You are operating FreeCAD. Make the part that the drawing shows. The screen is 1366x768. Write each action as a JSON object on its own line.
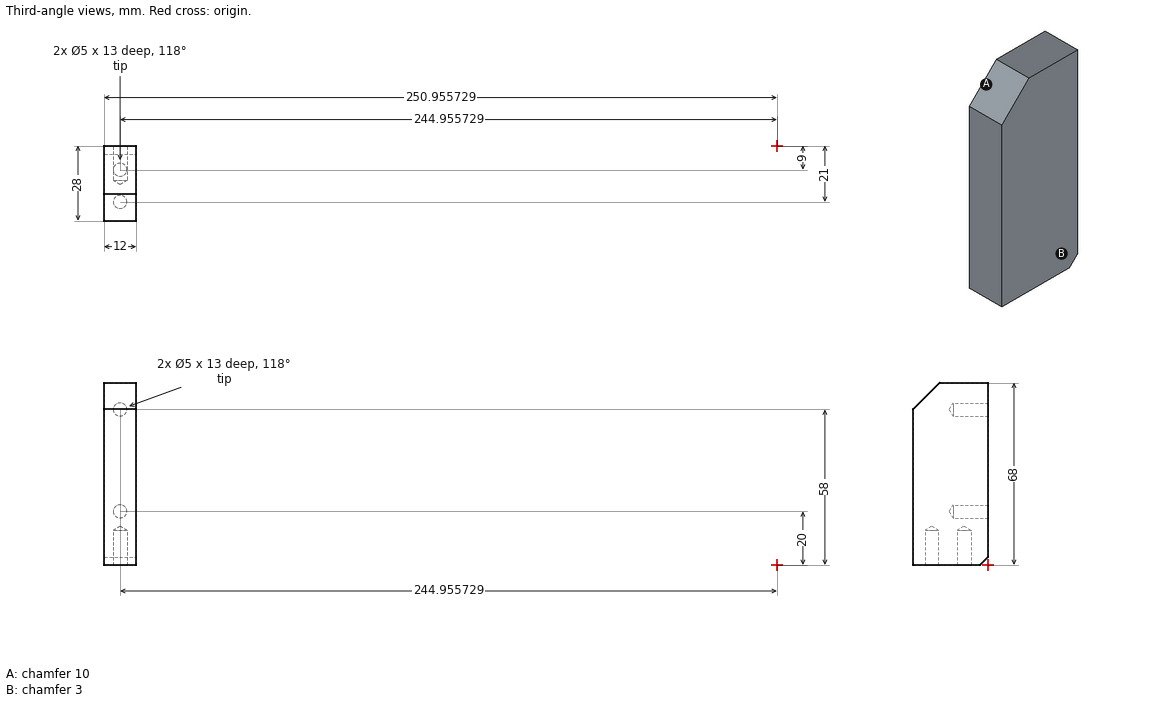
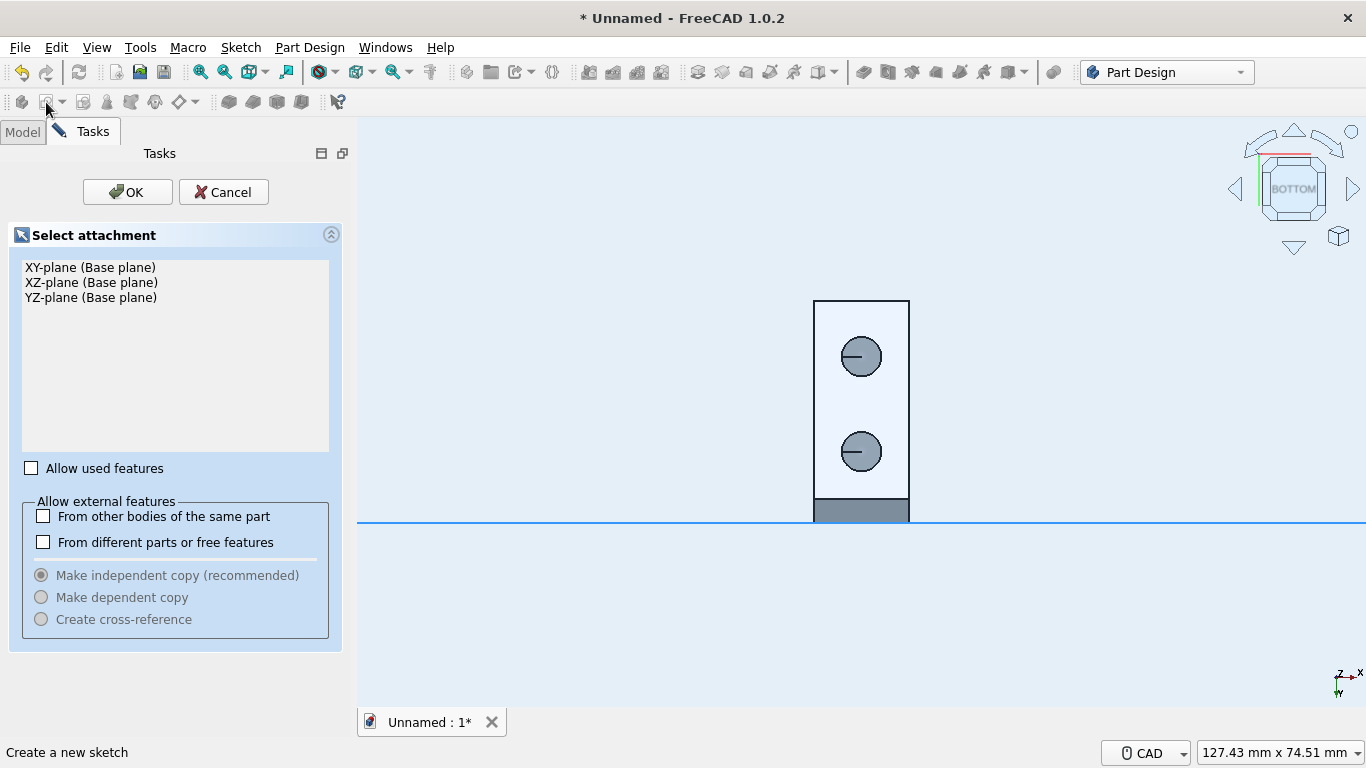
{"action": "left_click", "coordinate": [82, 282]}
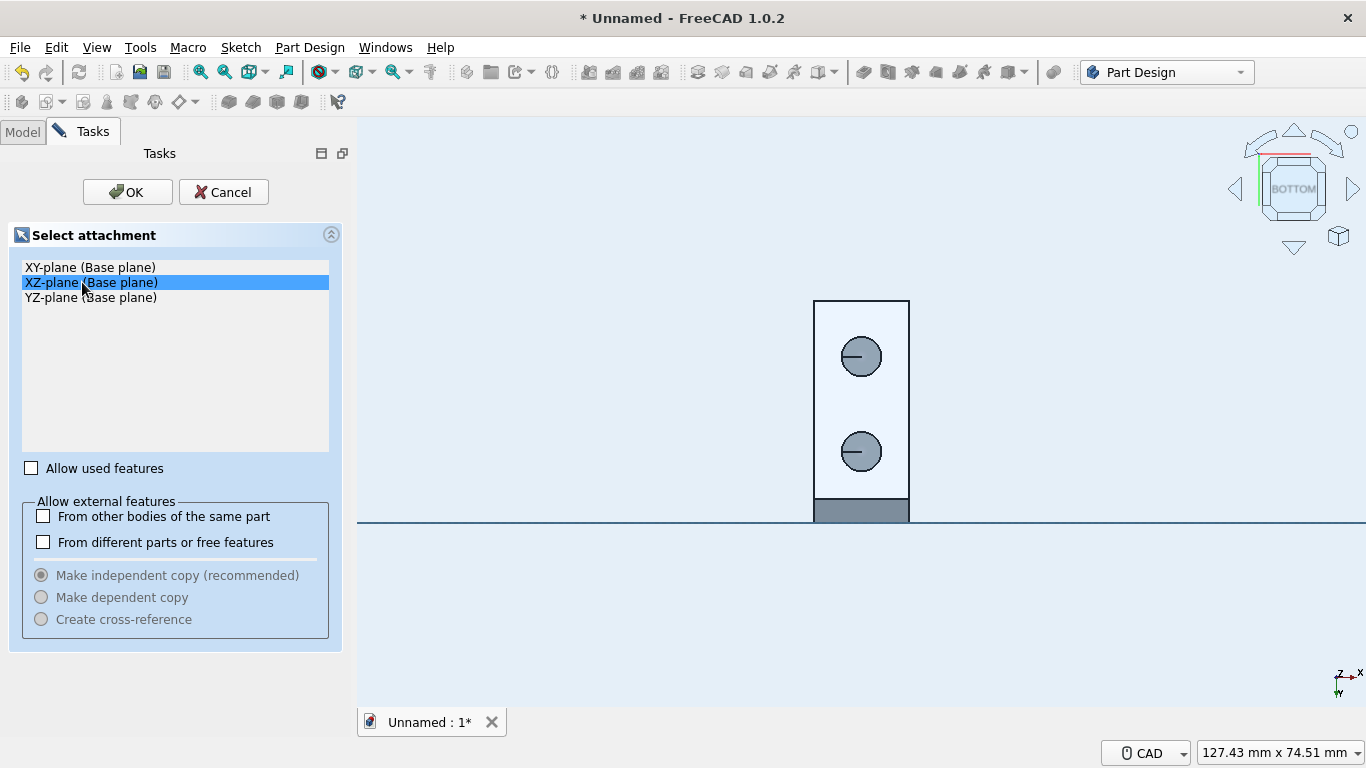
{"action": "left_click", "coordinate": [128, 192]}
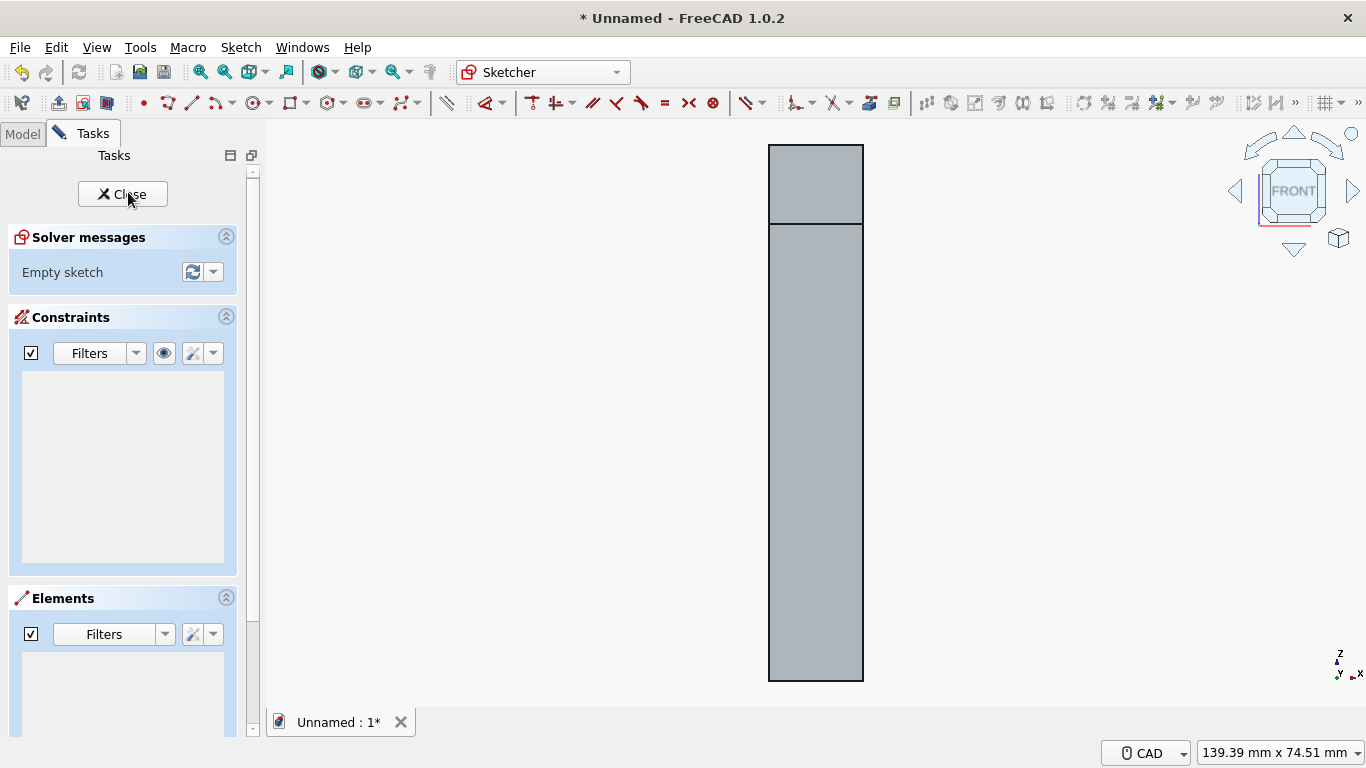
{"action": "left_click", "coordinate": [108, 104]}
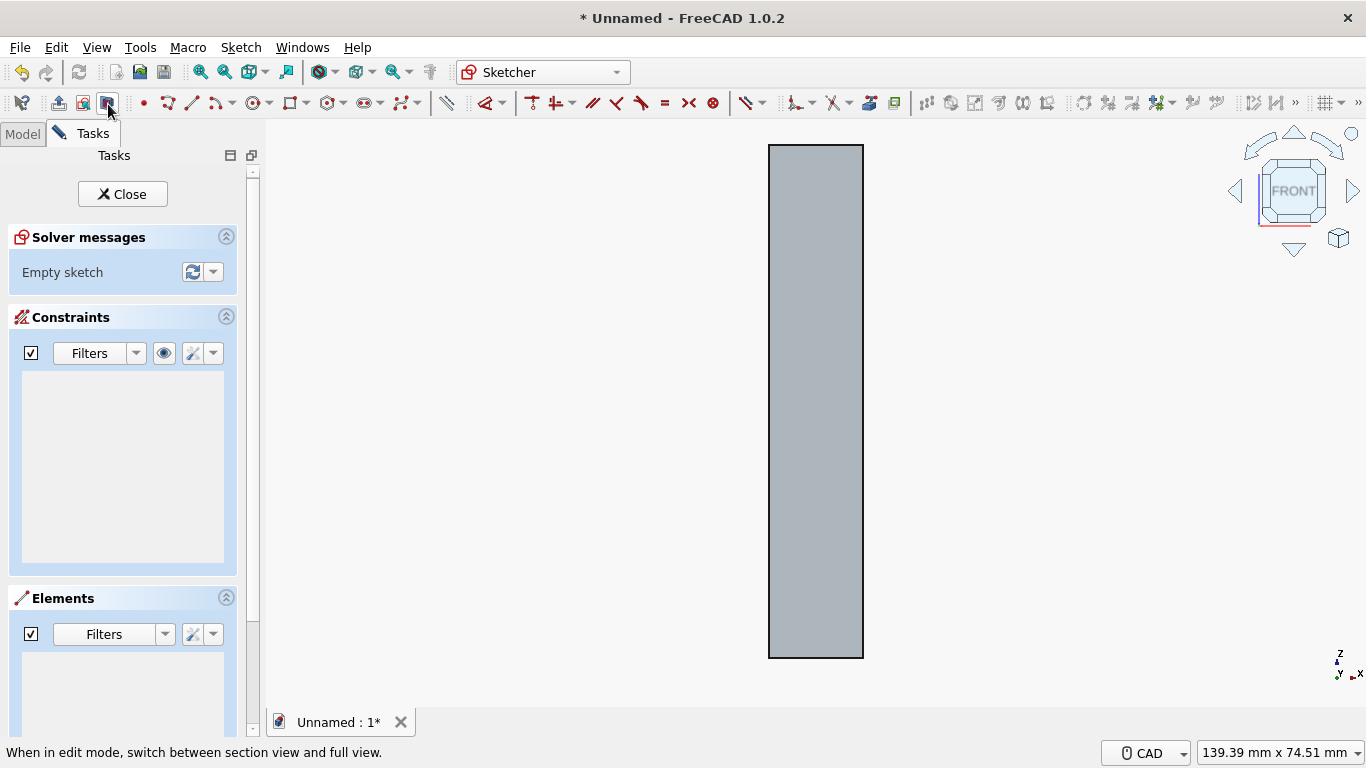
{"action": "left_click", "coordinate": [254, 104]}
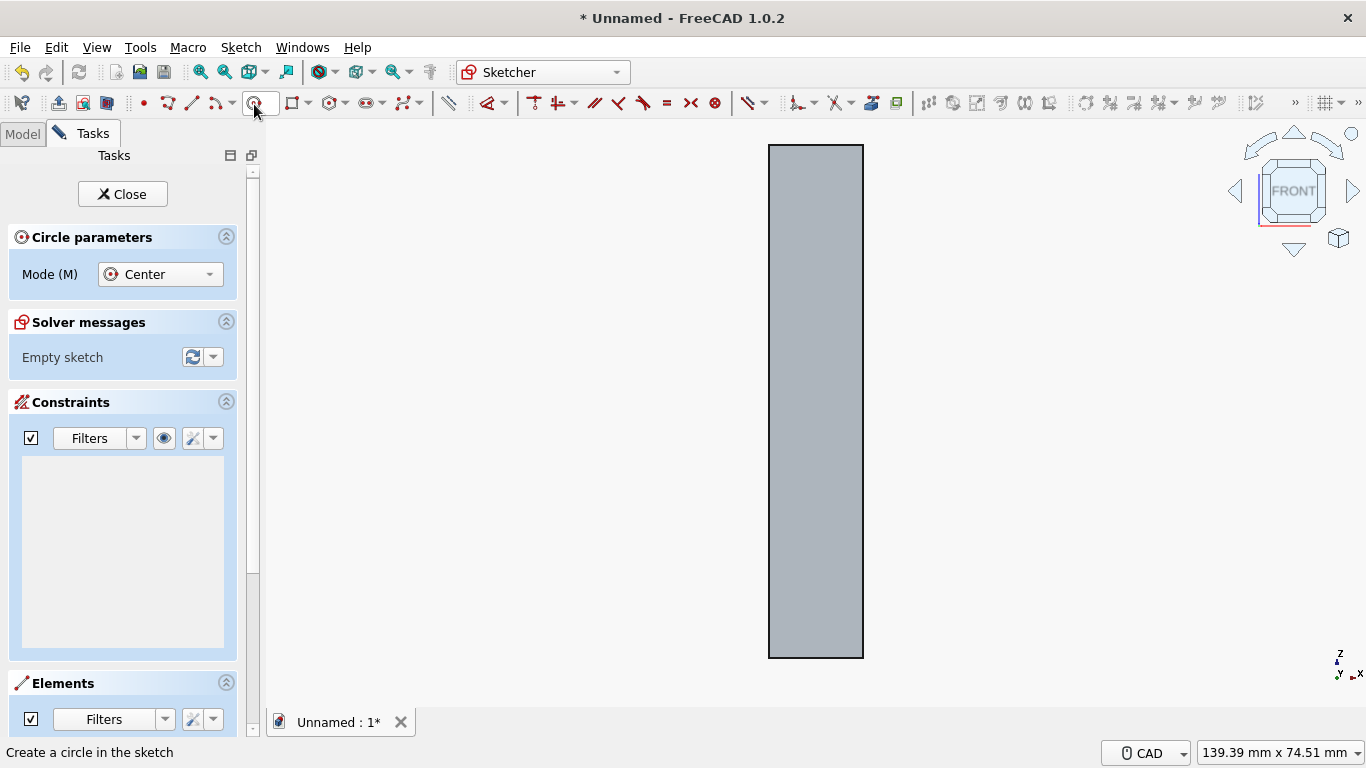
{"action": "left_click", "coordinate": [816, 224]}
{"action": "mouse_move", "coordinate": [830, 210]}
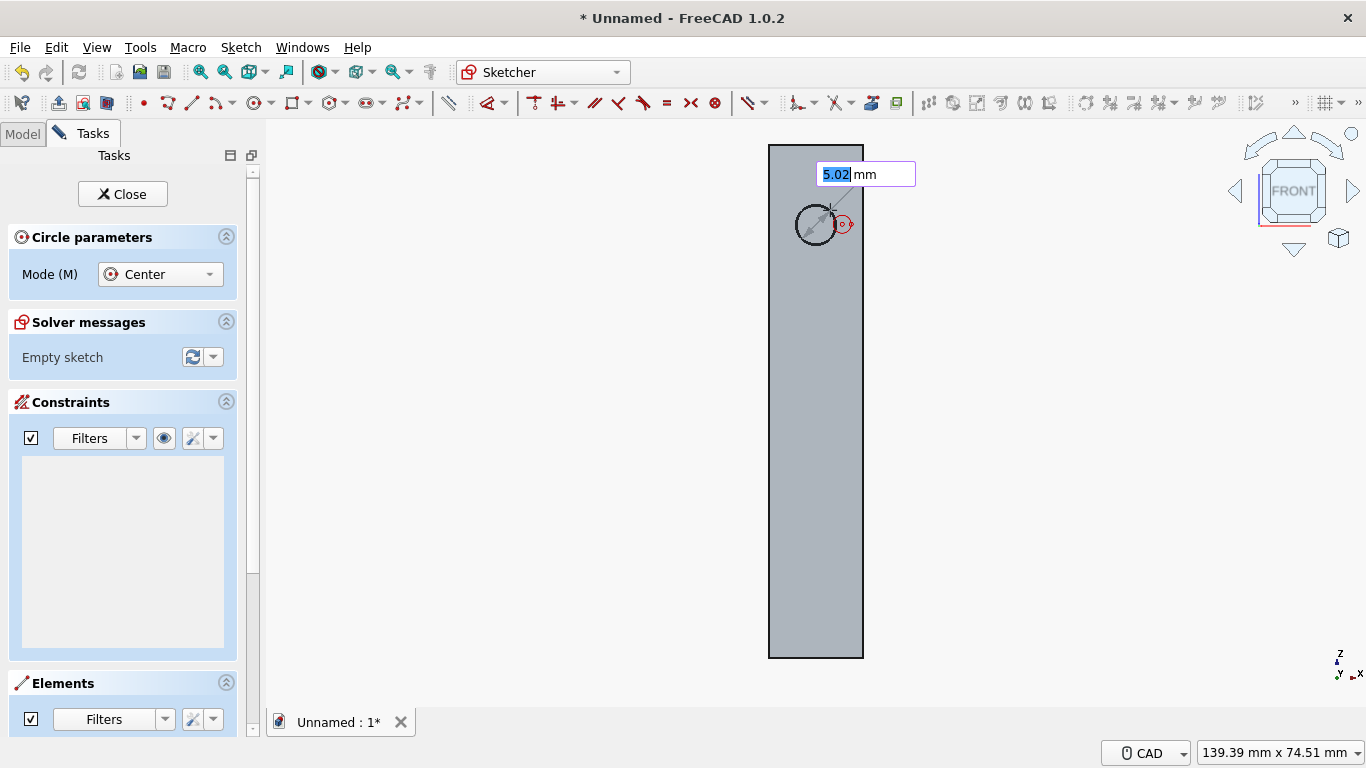
{"action": "type", "text": "5"}
{"action": "key", "text": "Return"}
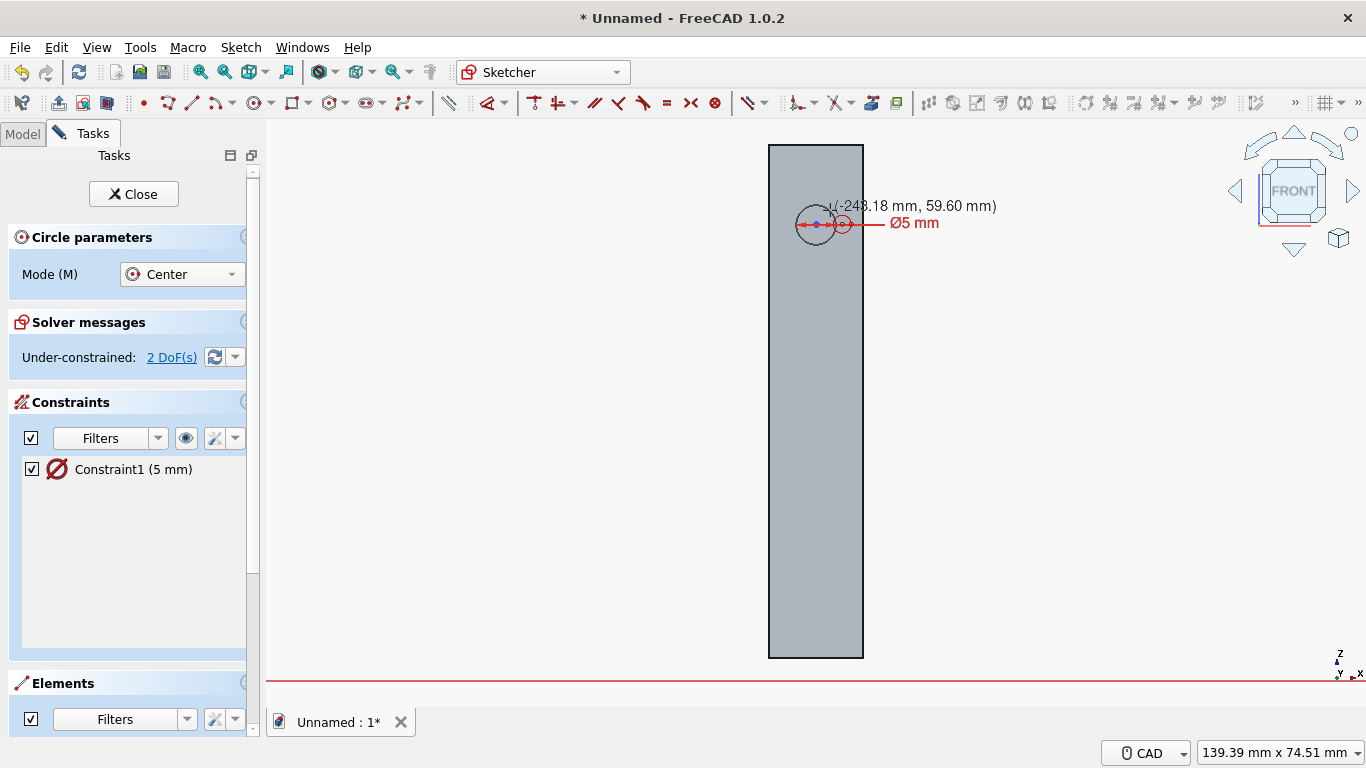
{"action": "left_click", "coordinate": [816, 523]}
{"action": "mouse_move", "coordinate": [830, 510]}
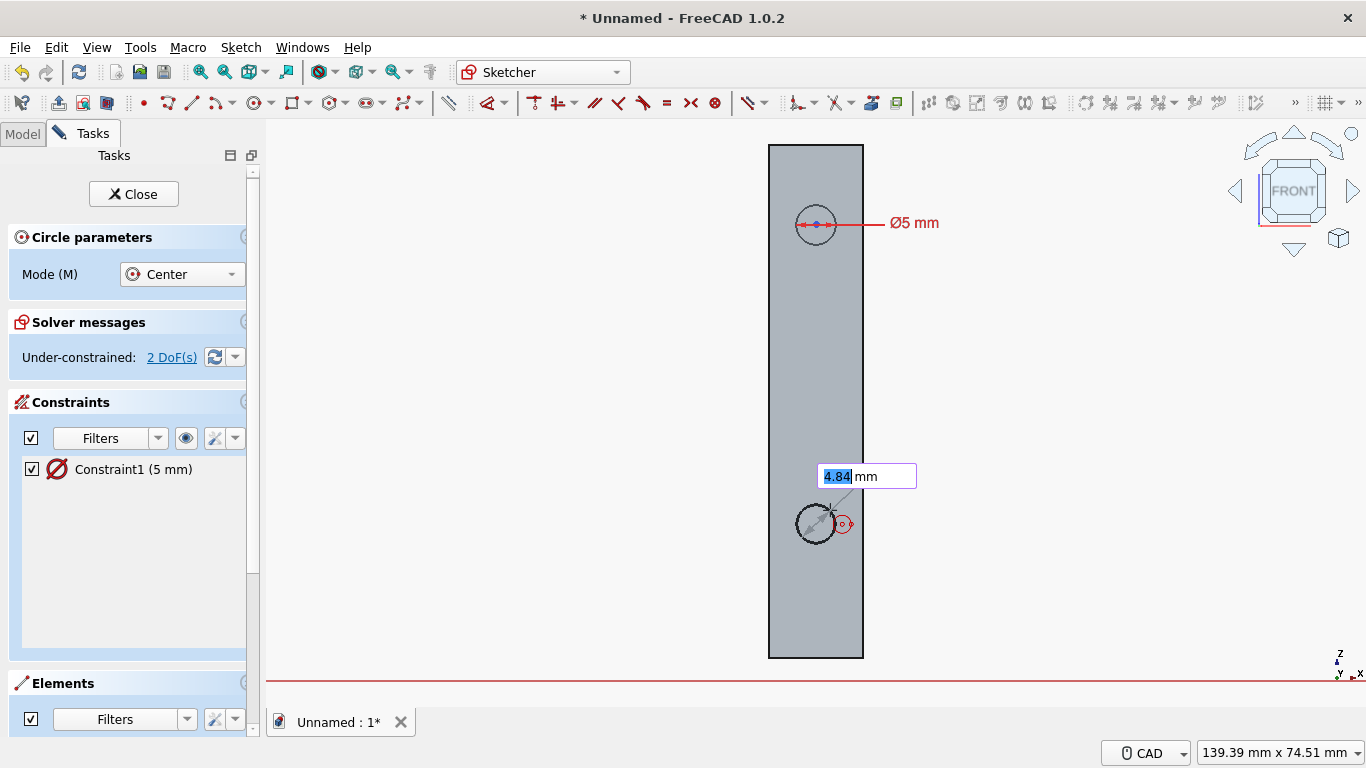
{"action": "type", "text": "5"}
{"action": "key", "text": "Return"}
{"action": "key", "text": "Escape"}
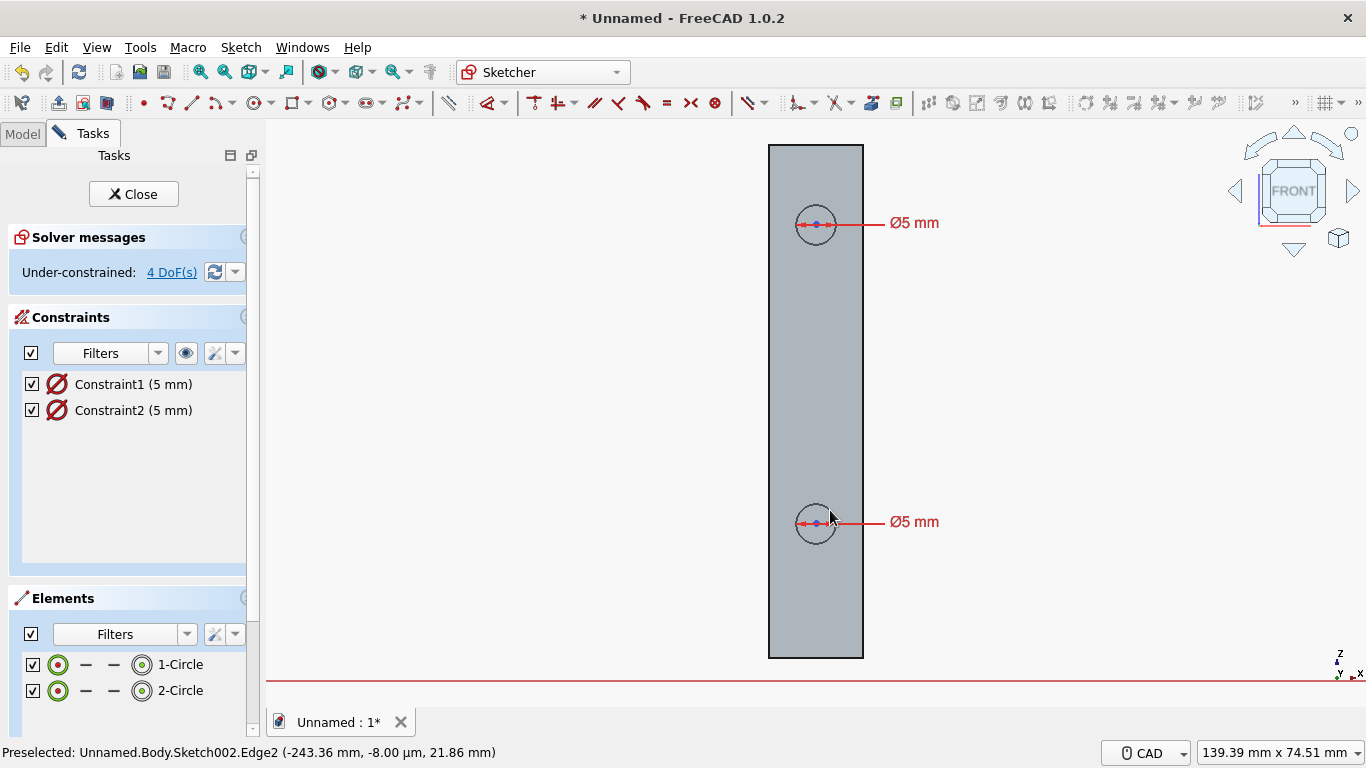
{"action": "left_click", "coordinate": [488, 104]}